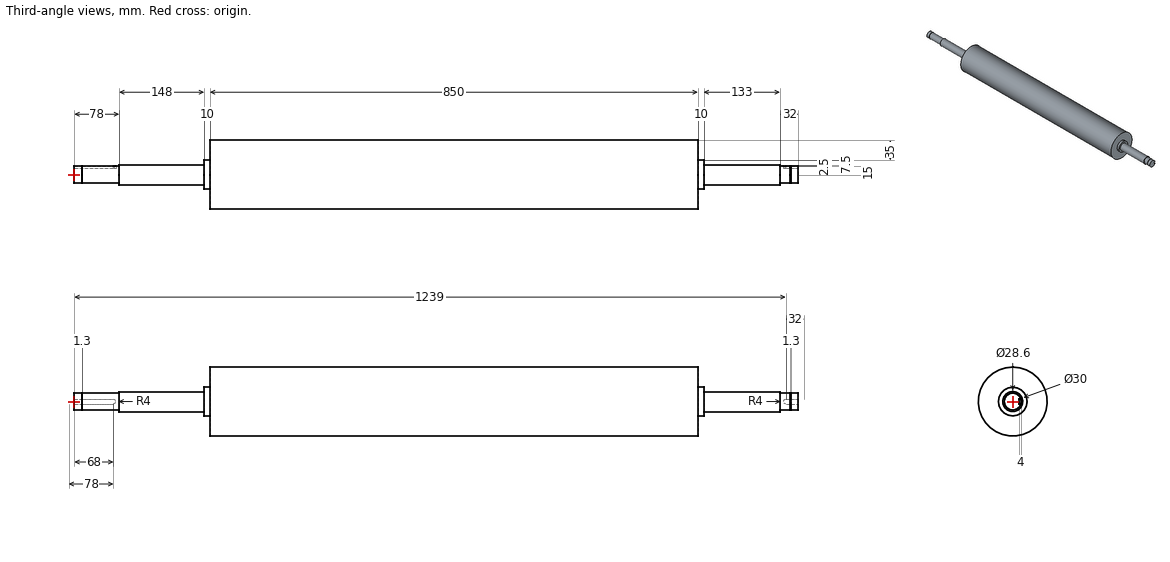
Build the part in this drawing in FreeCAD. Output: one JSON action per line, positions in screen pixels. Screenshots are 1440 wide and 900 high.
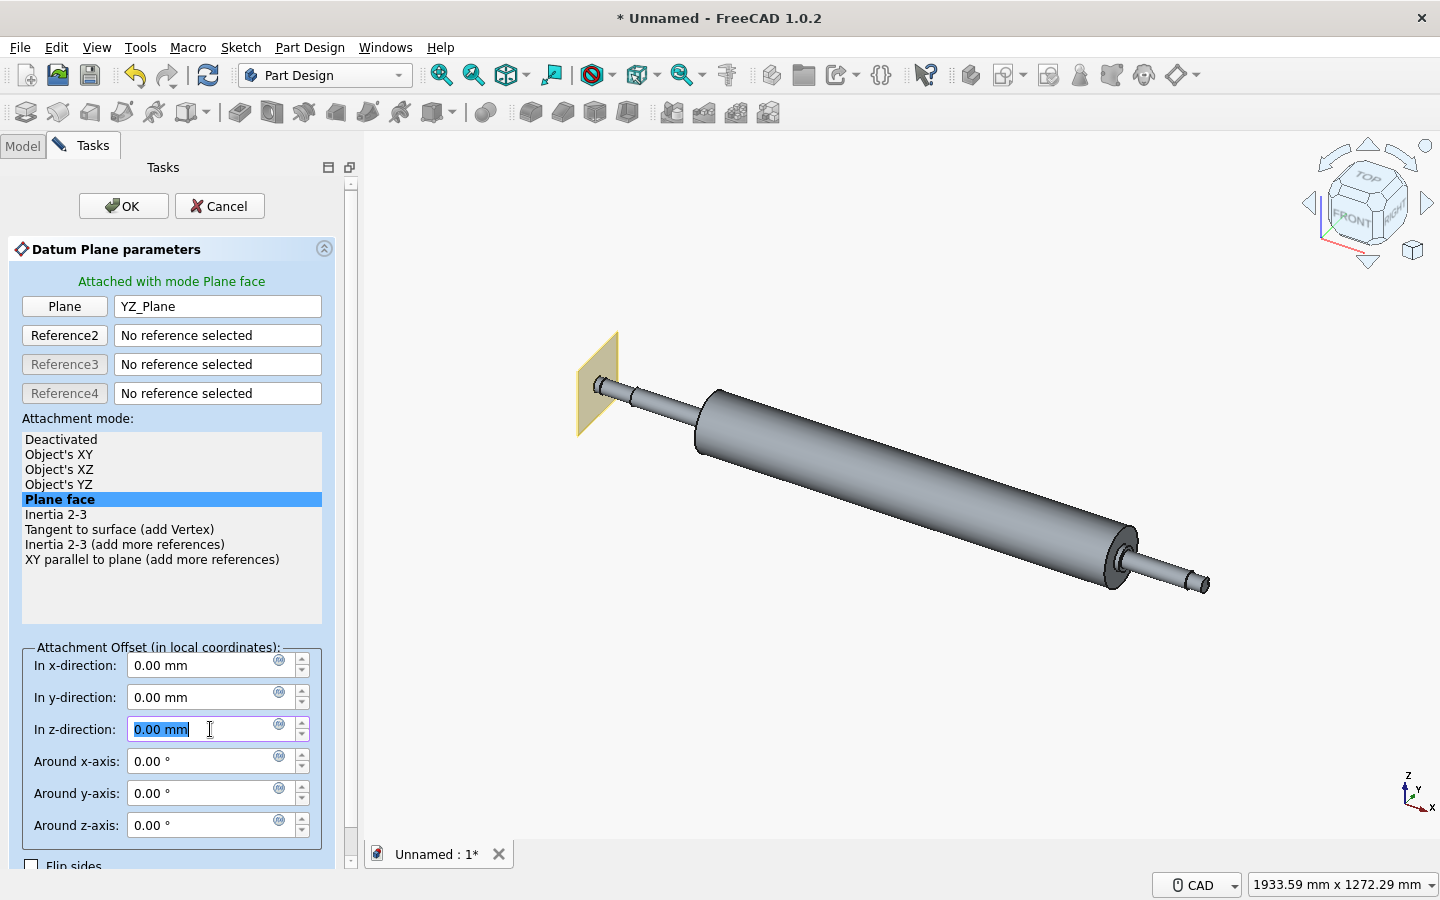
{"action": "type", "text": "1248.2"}
{"action": "key", "text": "Tab"}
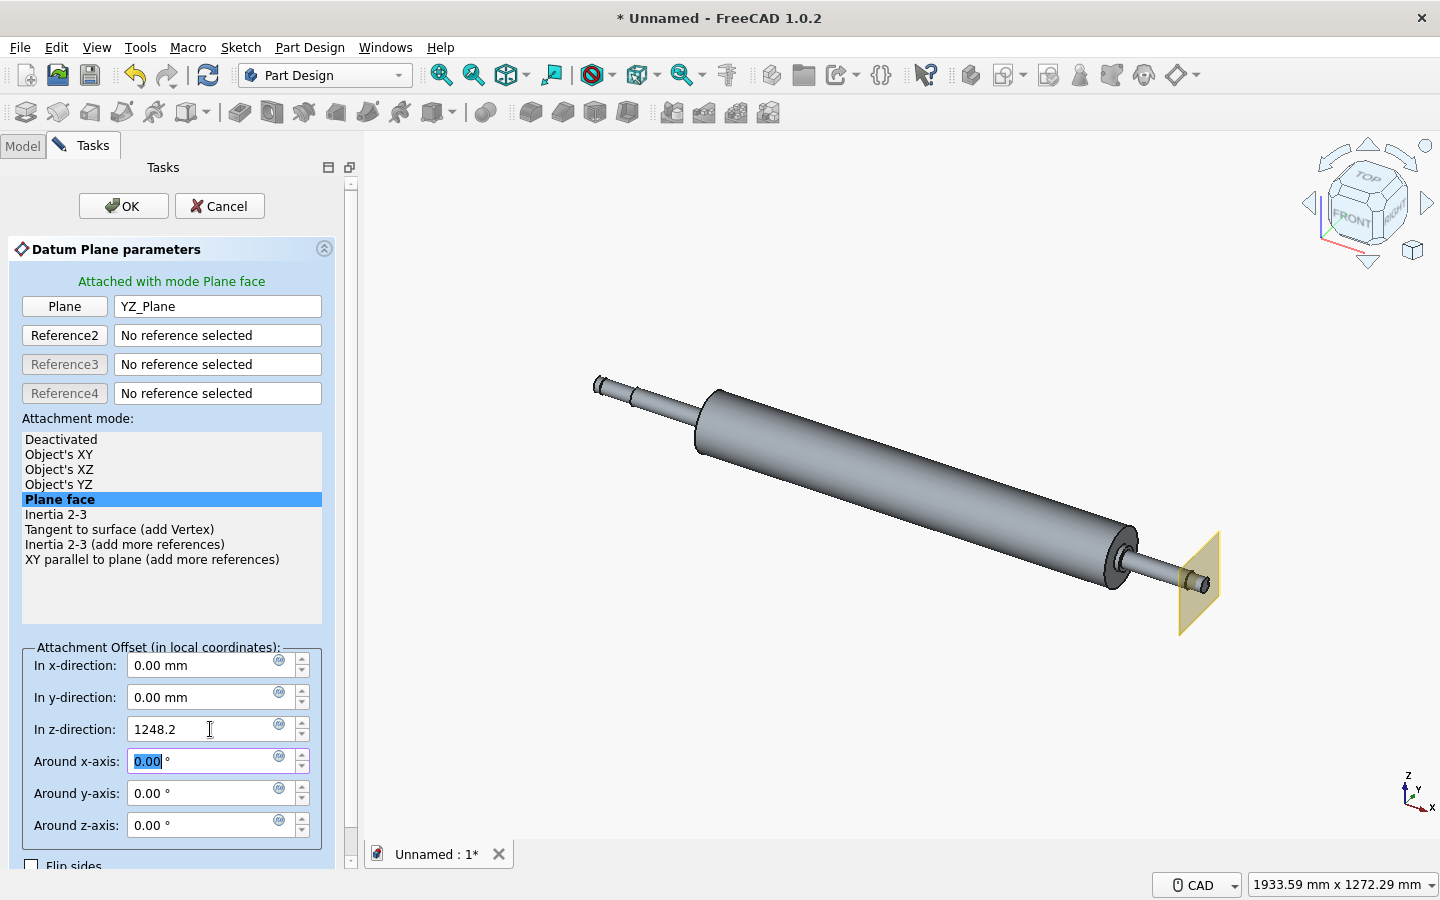
{"action": "left_click", "coordinate": [124, 206]}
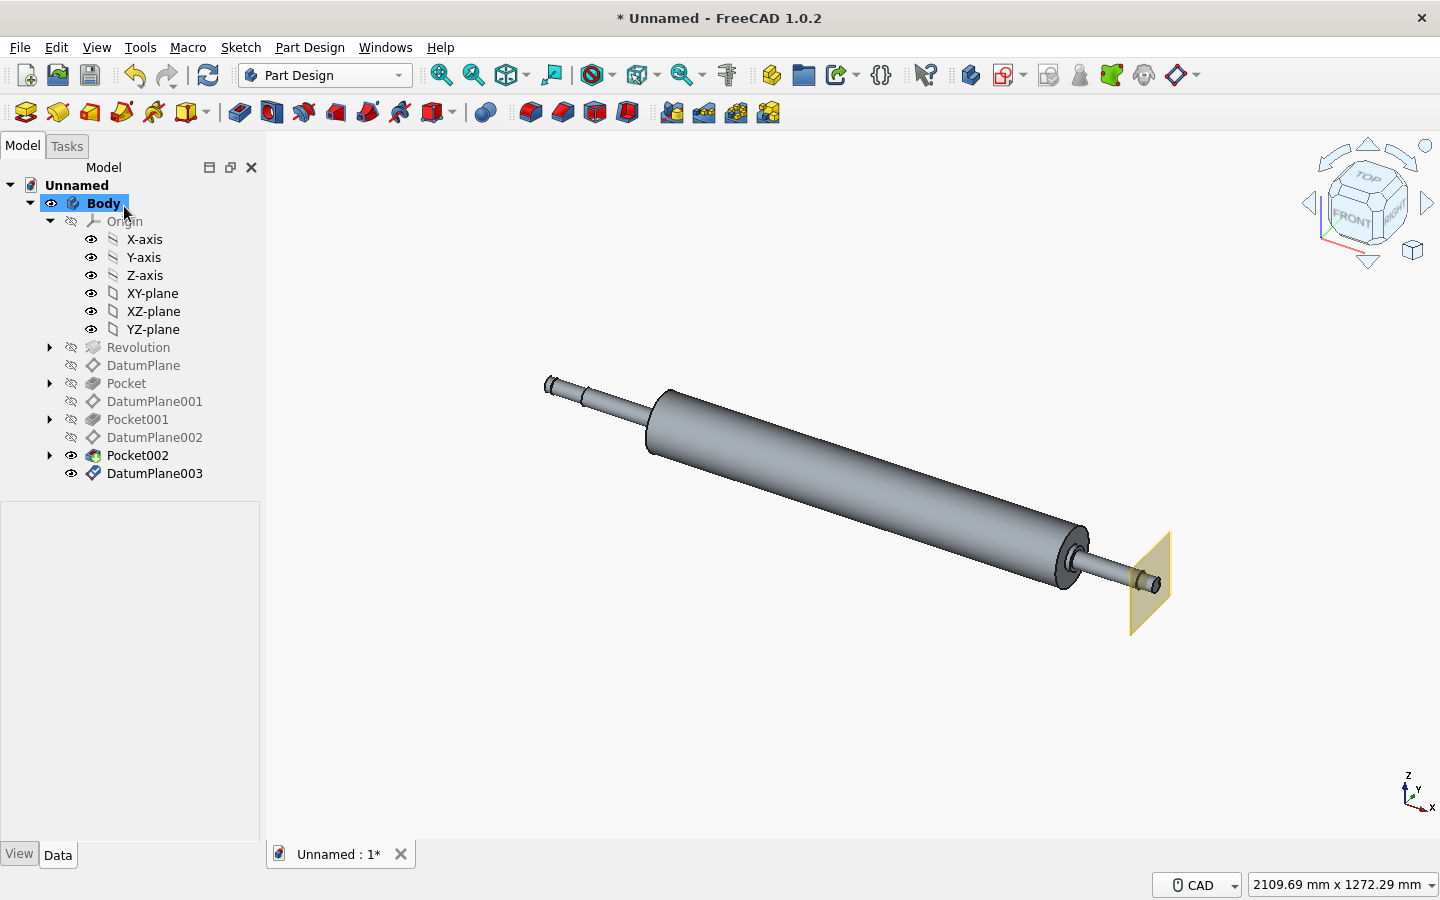
{"action": "left_click", "coordinate": [116, 473]}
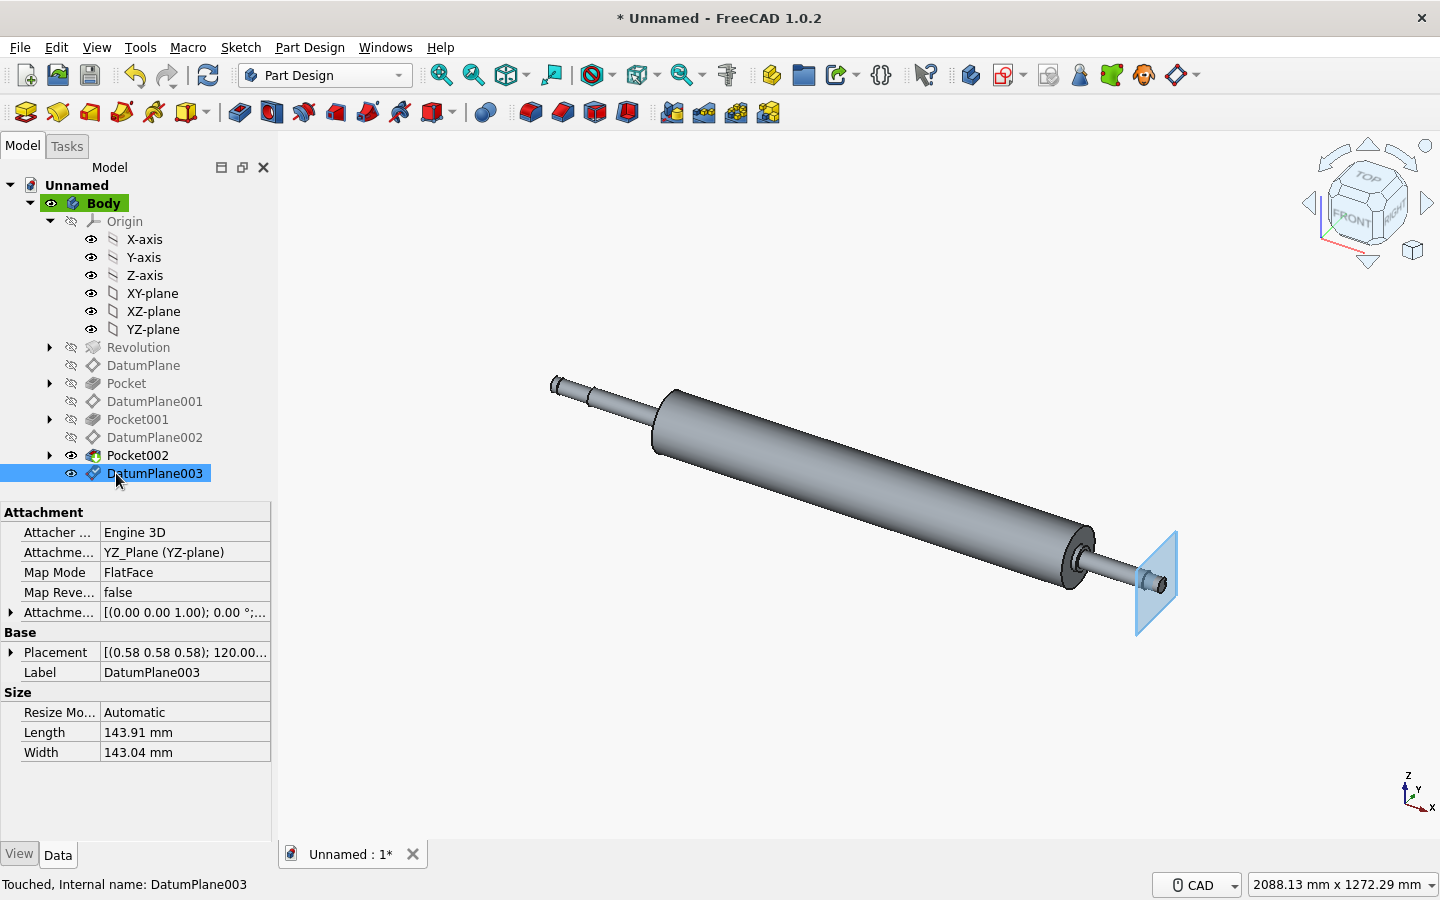
{"action": "left_click", "coordinate": [1004, 76]}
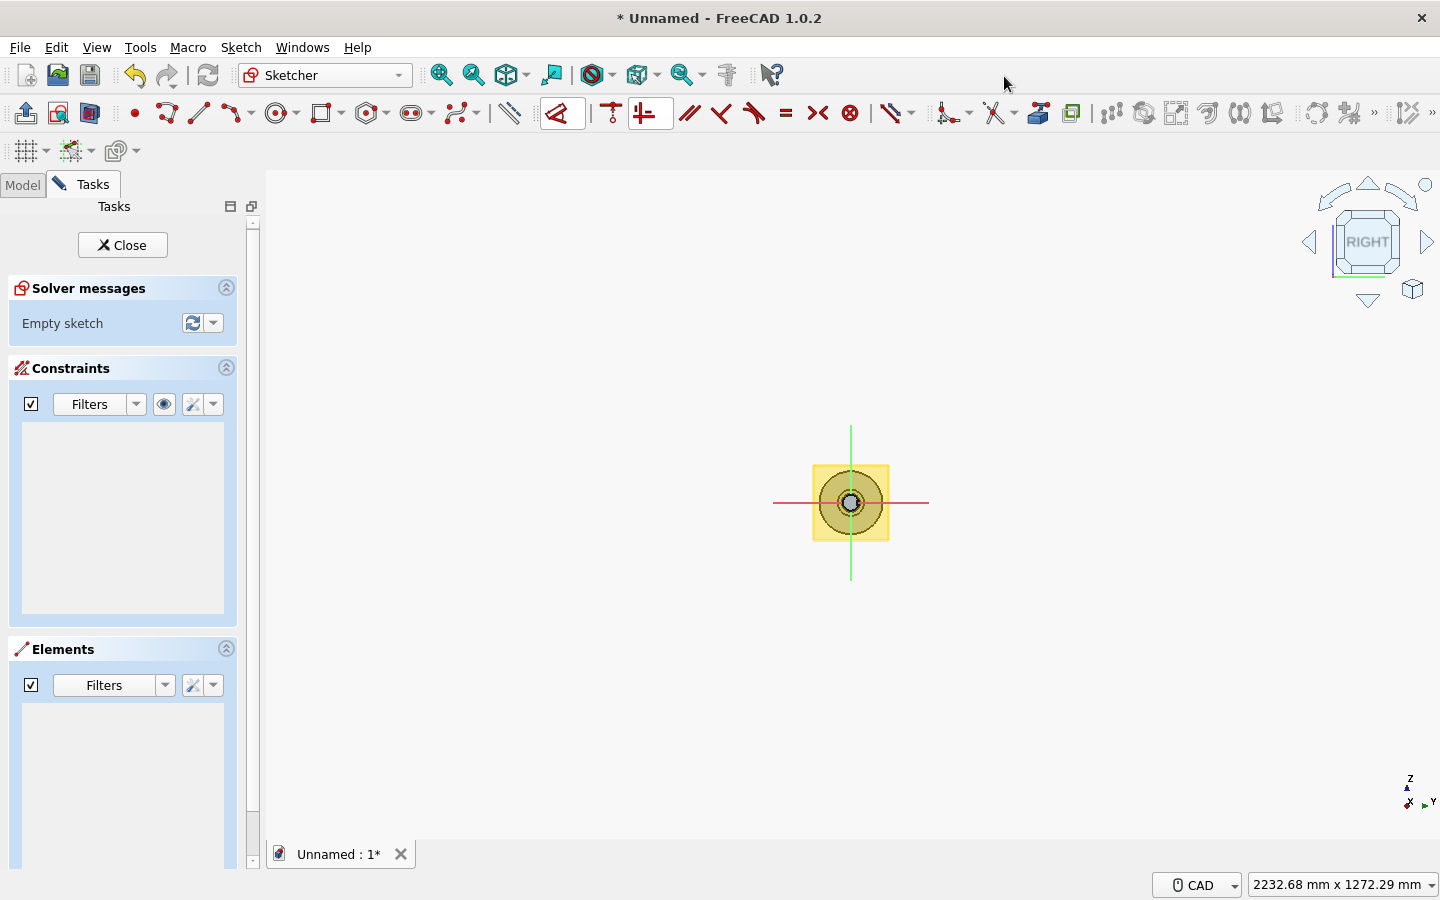
{"action": "left_click", "coordinate": [90, 114]}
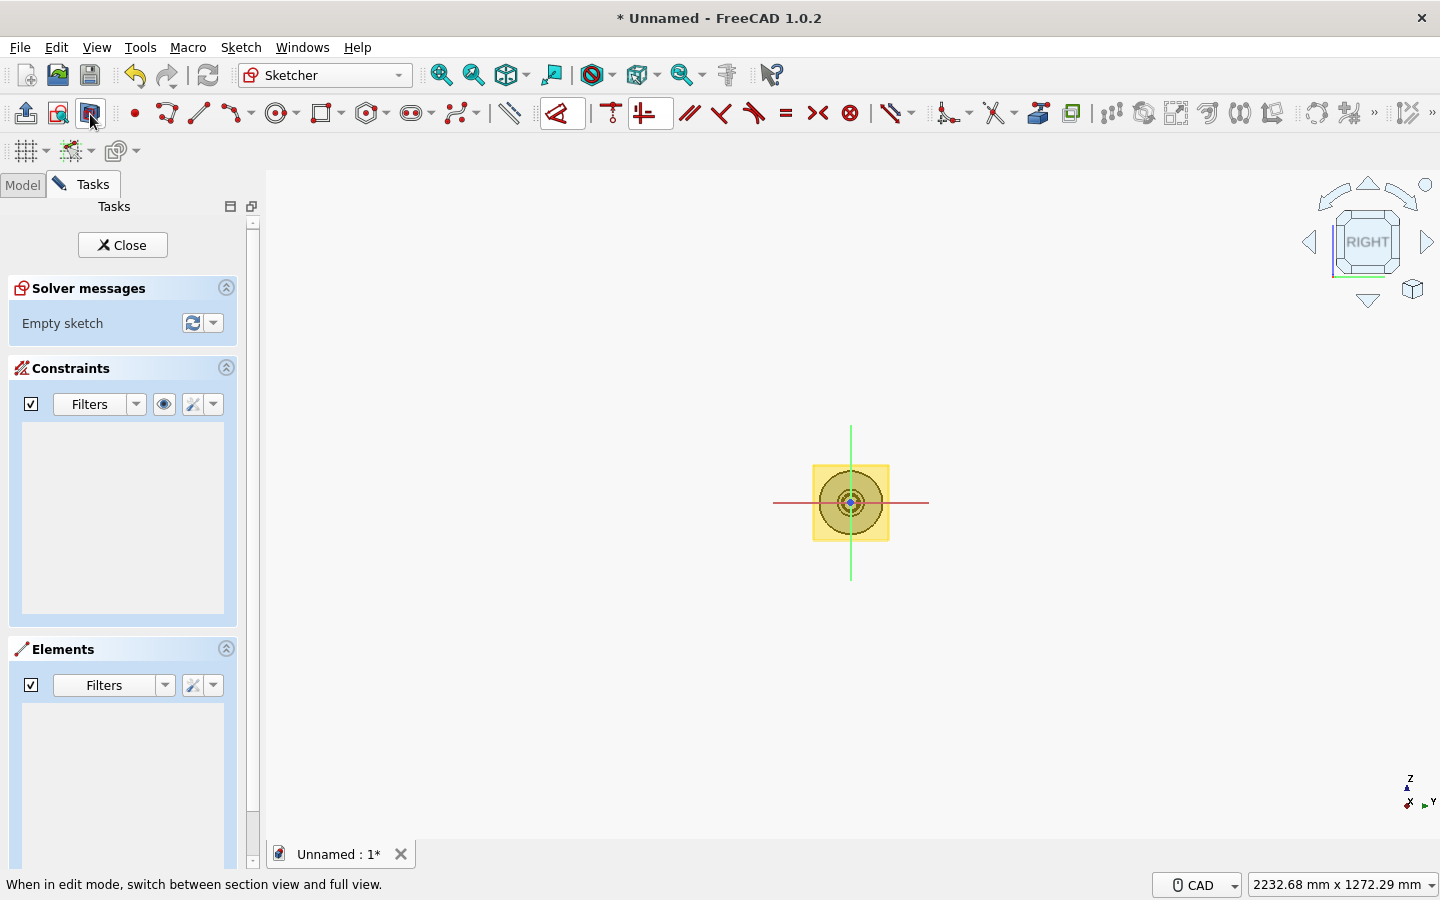
{"action": "scroll", "coordinate": [854, 503], "scroll_direction": "up", "scroll_amount": 15}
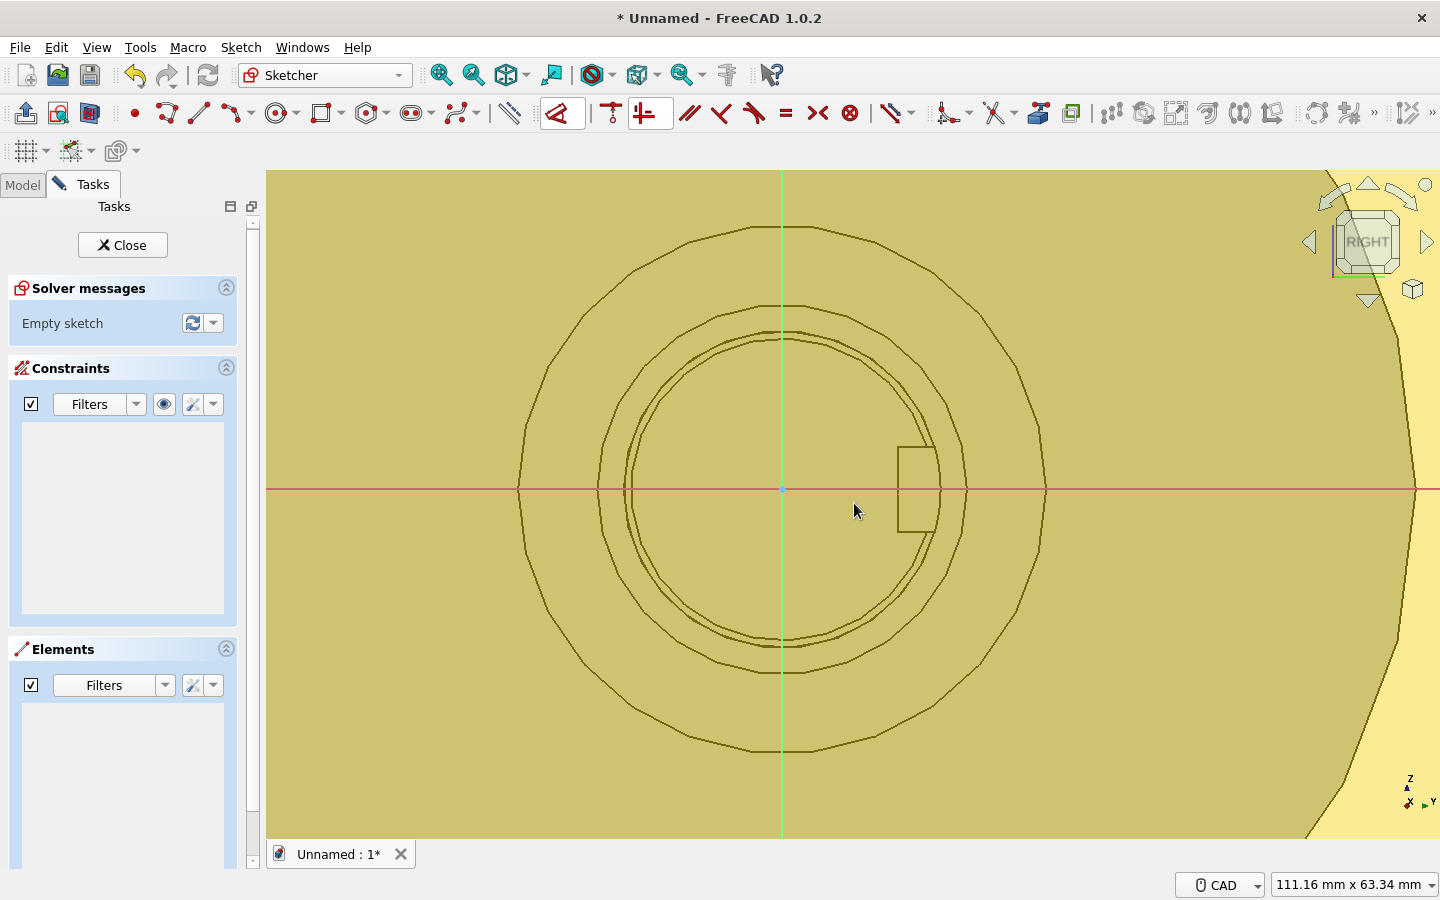
{"action": "scroll", "coordinate": [777, 459], "scroll_direction": "up", "scroll_amount": 2}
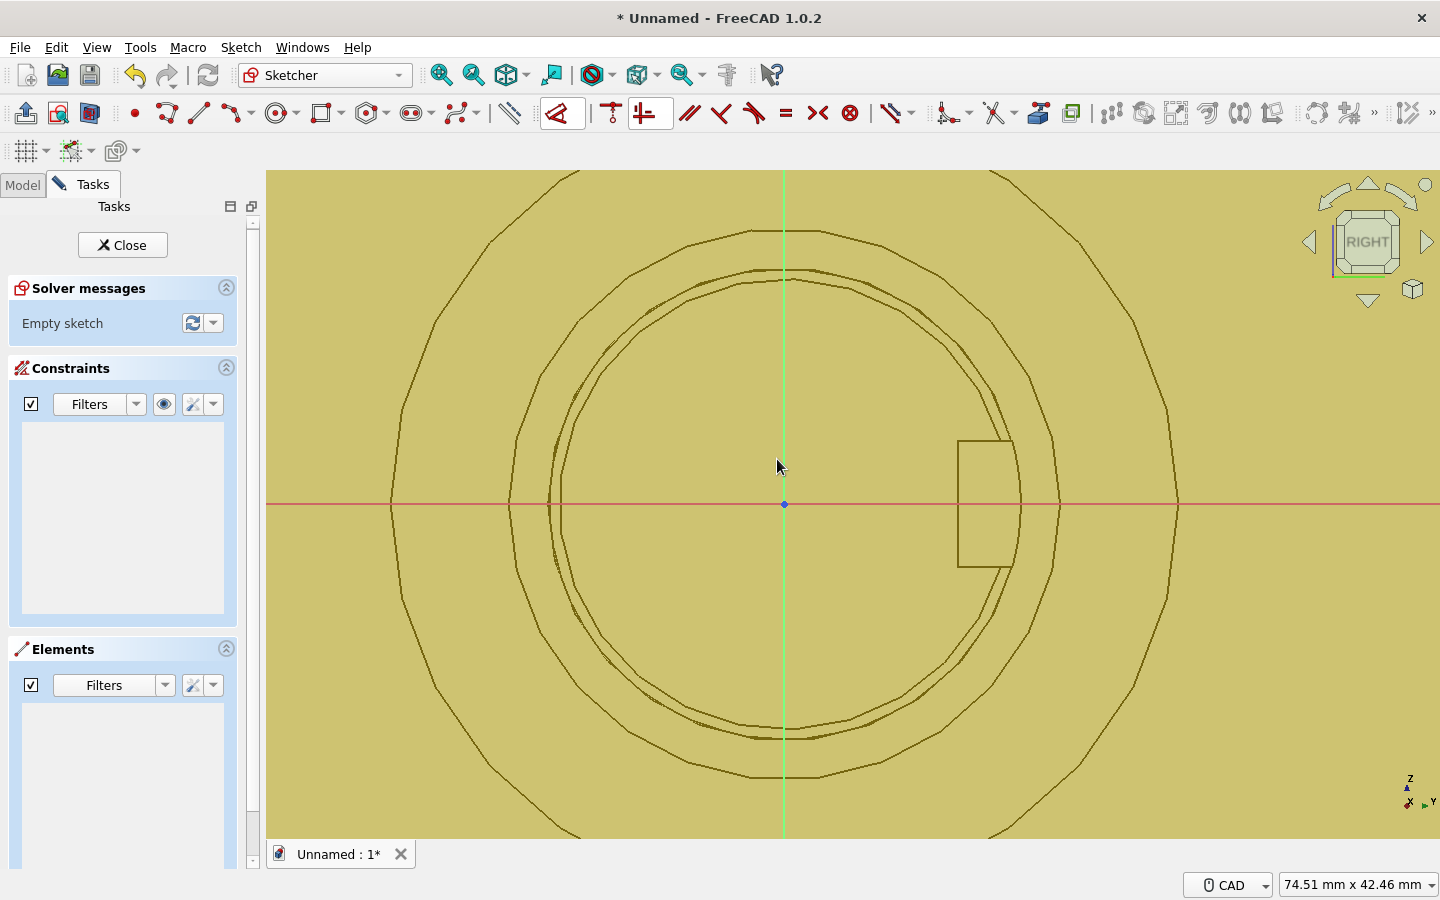
{"action": "left_click", "coordinate": [276, 114]}